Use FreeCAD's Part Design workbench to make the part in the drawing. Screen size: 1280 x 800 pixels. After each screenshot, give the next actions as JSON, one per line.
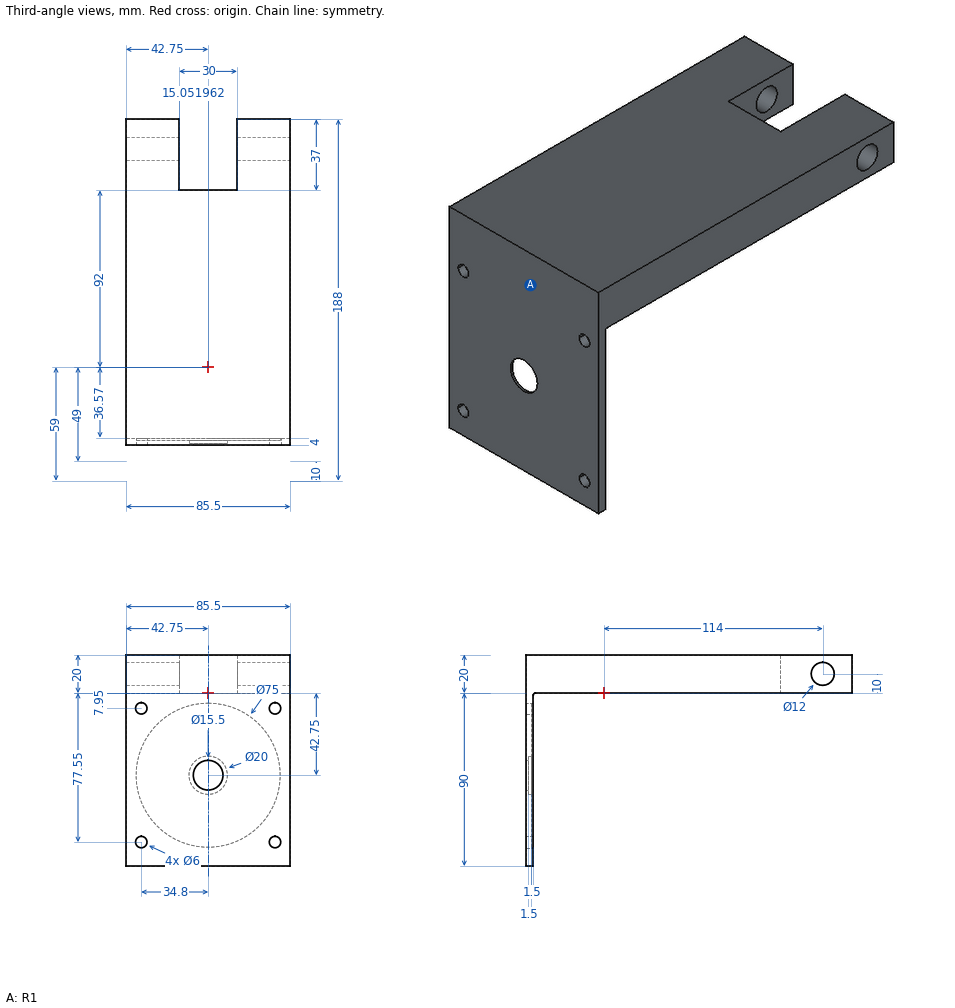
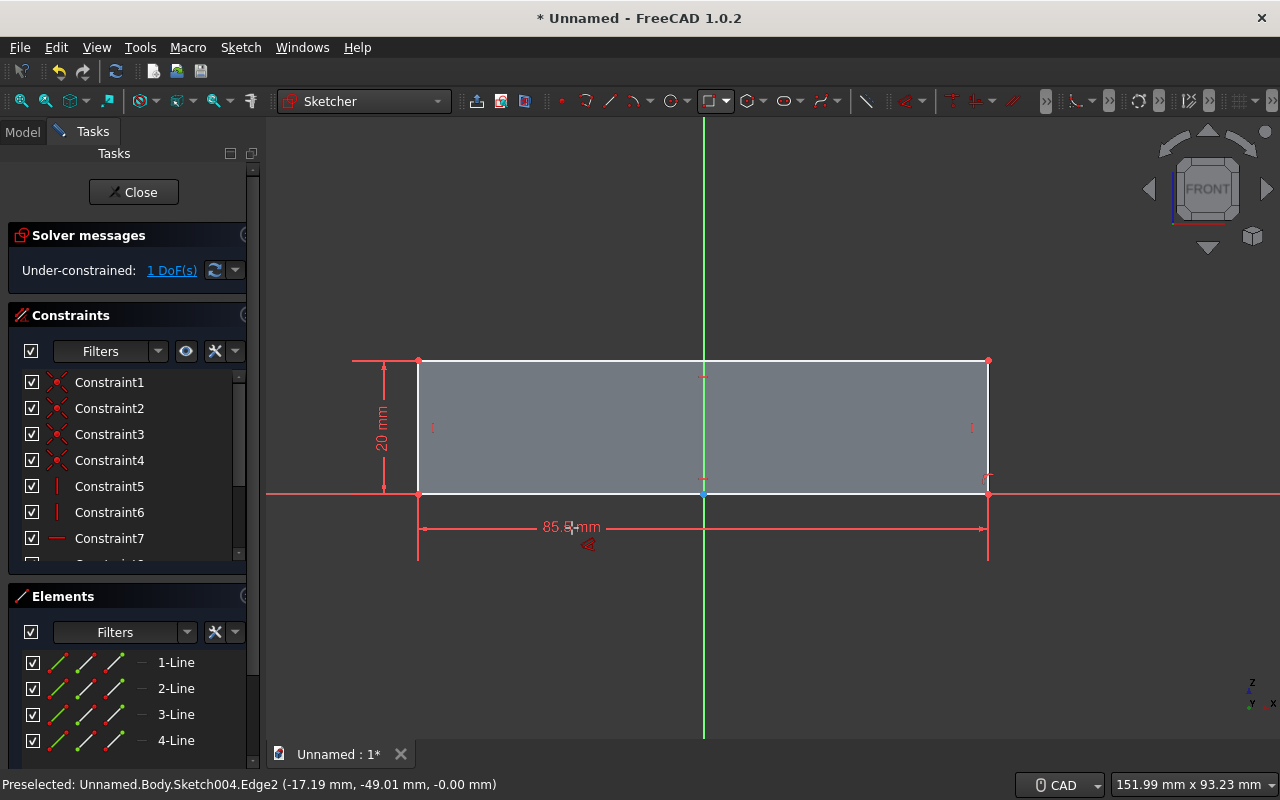
{"action": "left_click", "coordinate": [418, 361]}
{"action": "left_click", "coordinate": [495, 528]}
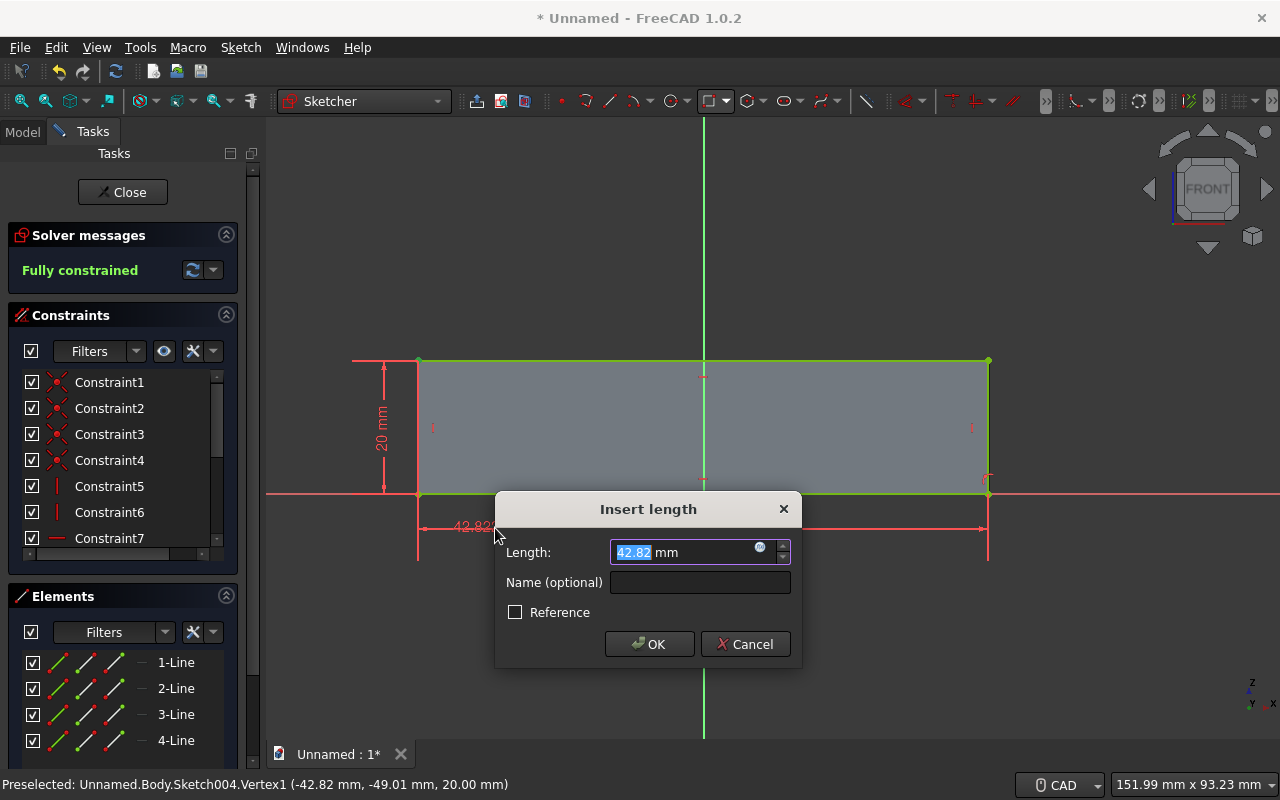
{"action": "type", "text": "42.75"}
{"action": "key", "text": "Return"}
{"action": "key", "text": "Escape"}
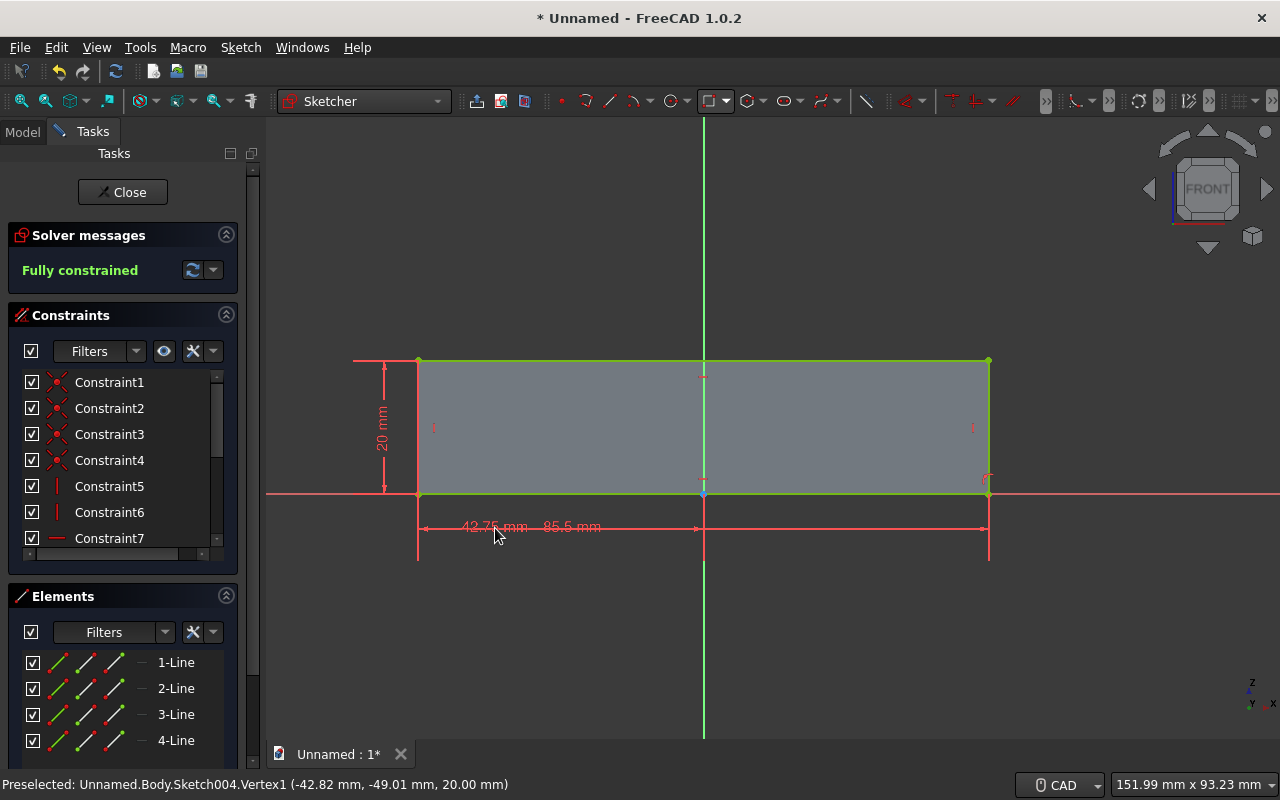
{"action": "left_click", "coordinate": [123, 192]}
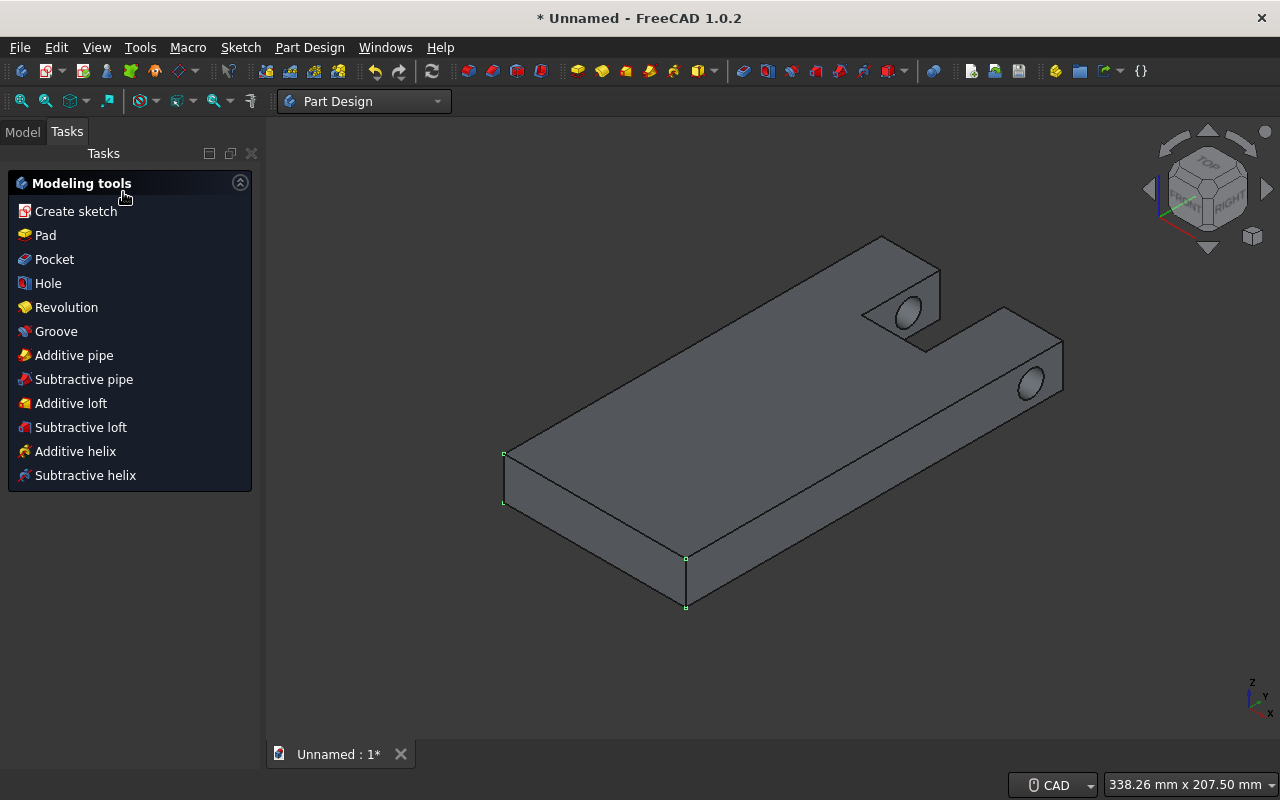
{"action": "left_click", "coordinate": [744, 72]}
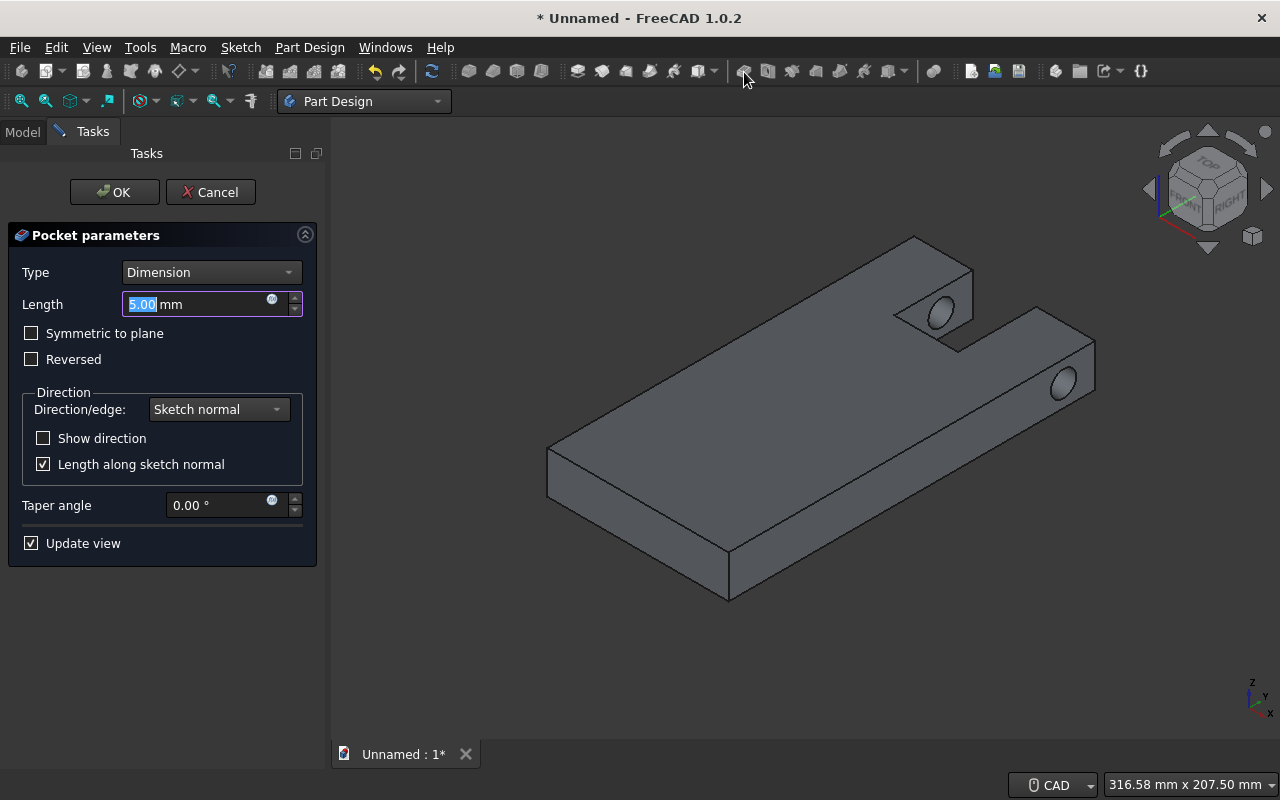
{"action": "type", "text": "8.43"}
{"action": "key", "text": "Tab"}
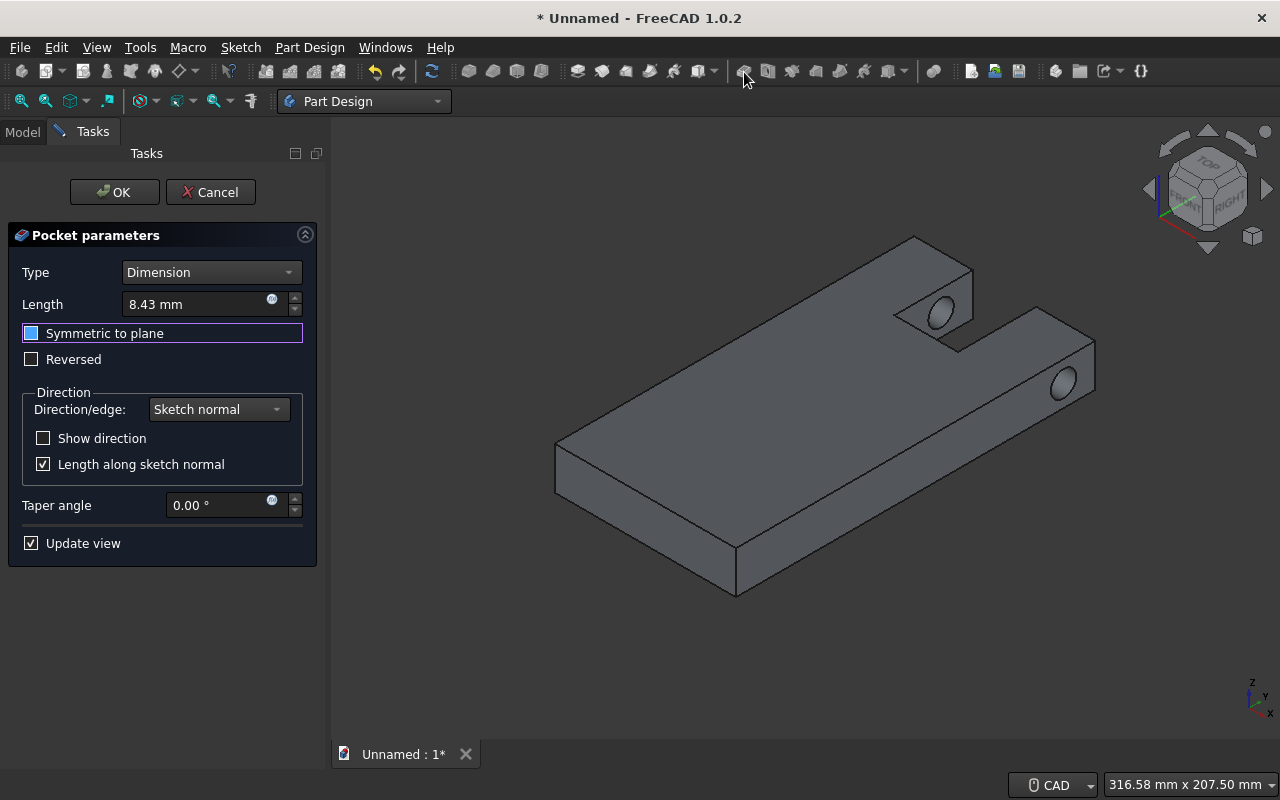
{"action": "left_click", "coordinate": [115, 192]}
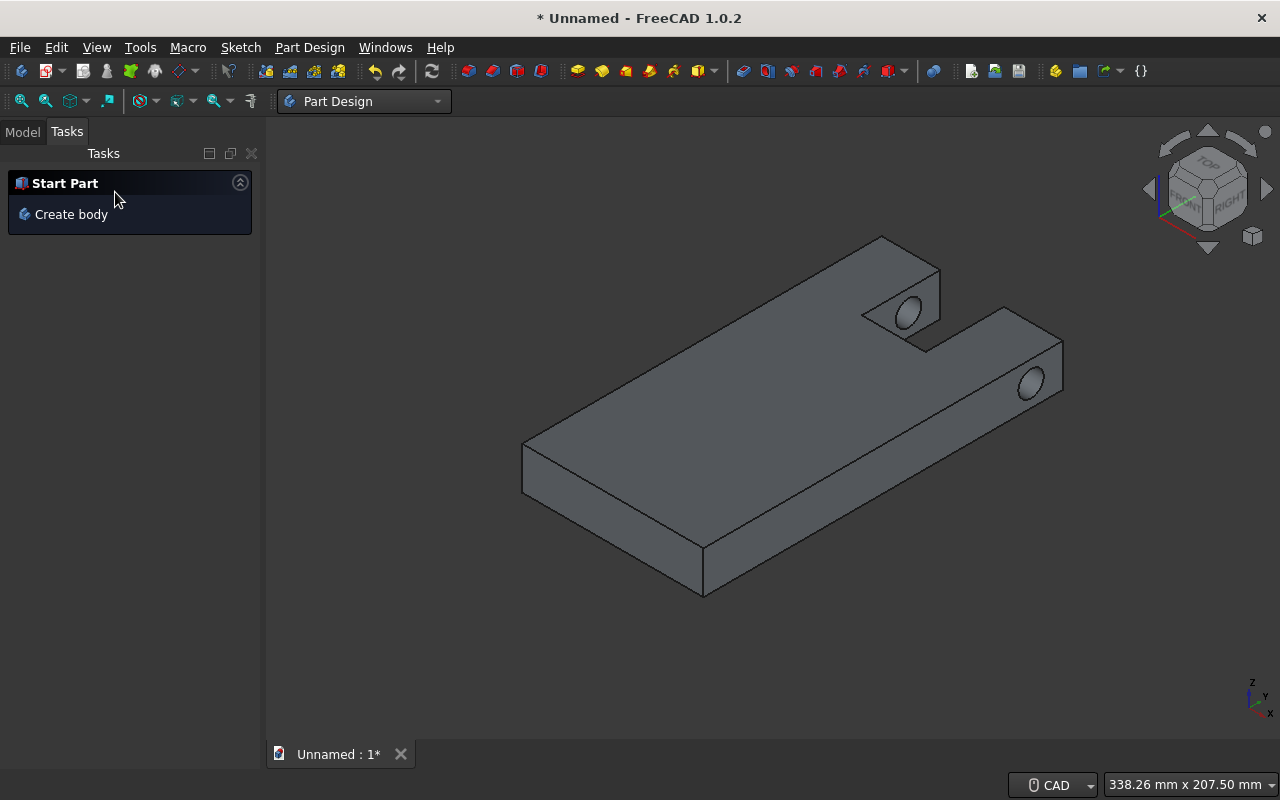
{"action": "left_click", "coordinate": [46, 72]}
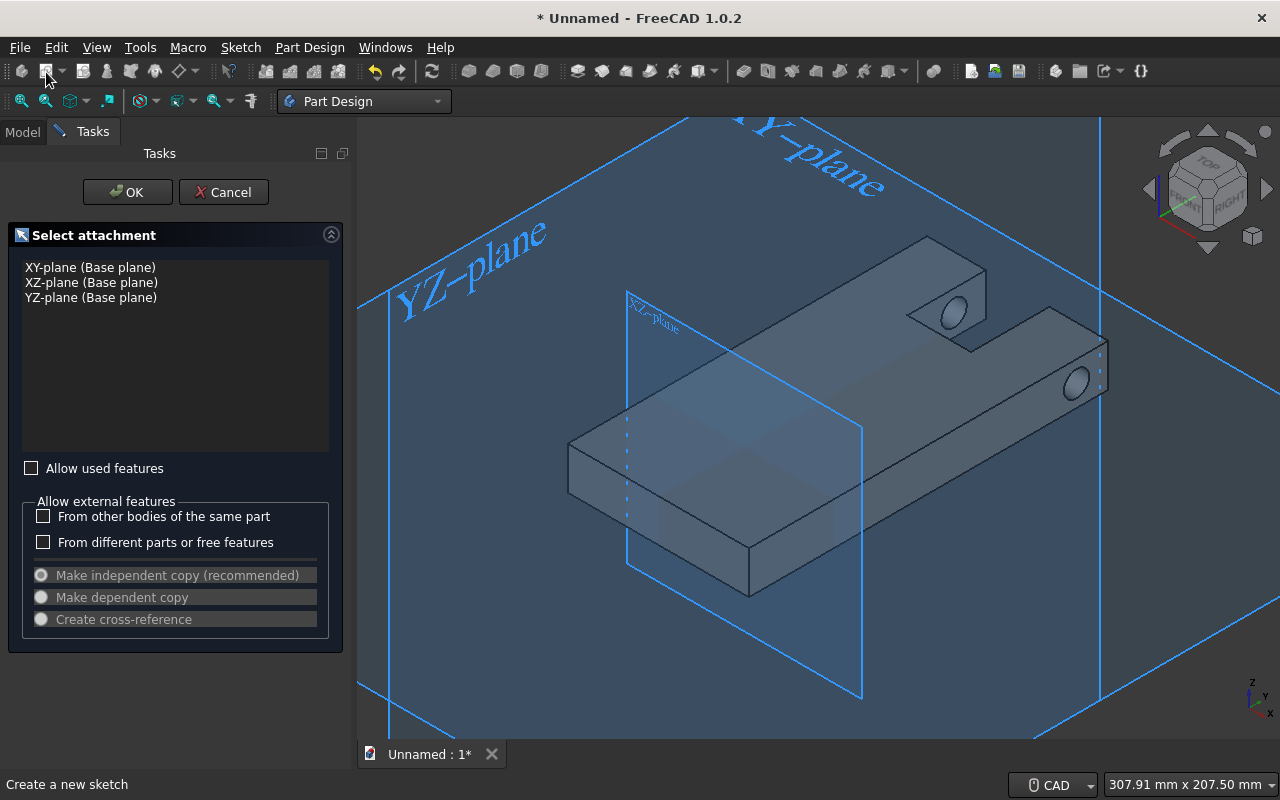
{"action": "left_click", "coordinate": [82, 268]}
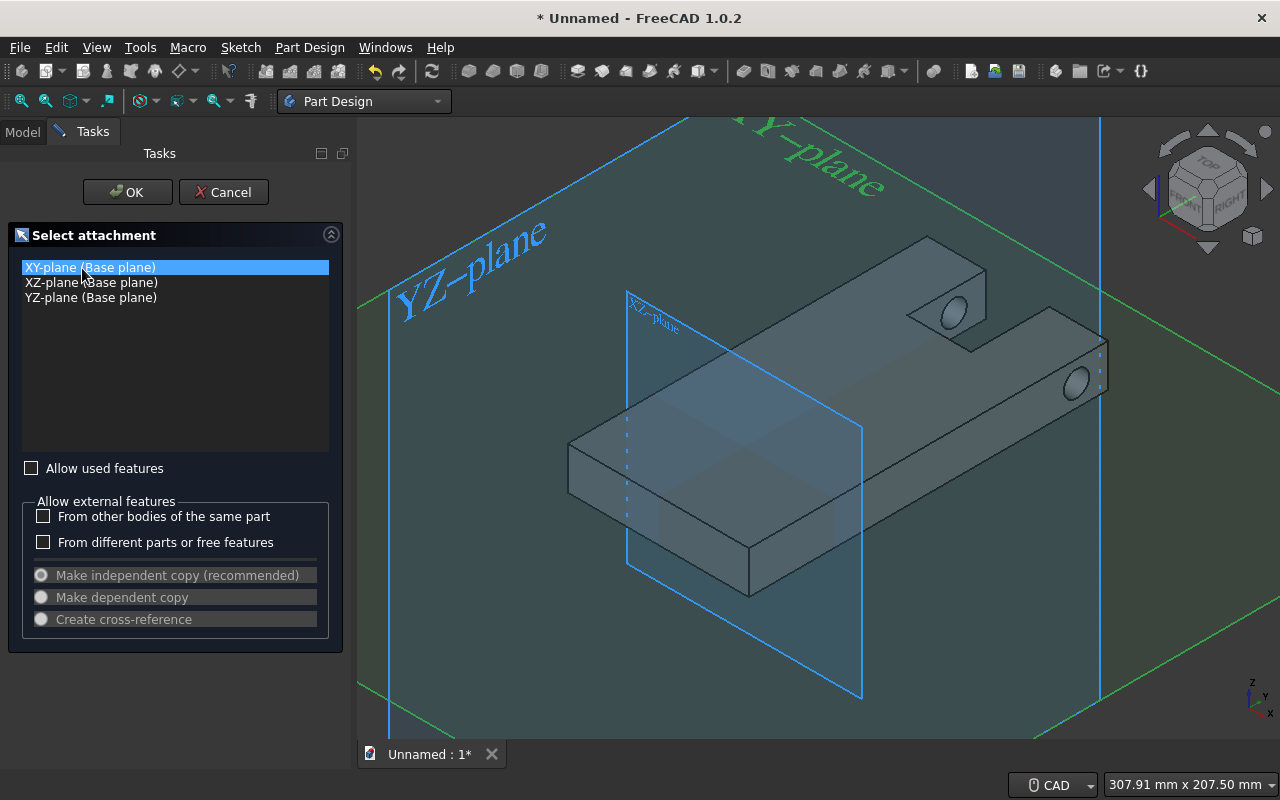
{"action": "left_click", "coordinate": [128, 192]}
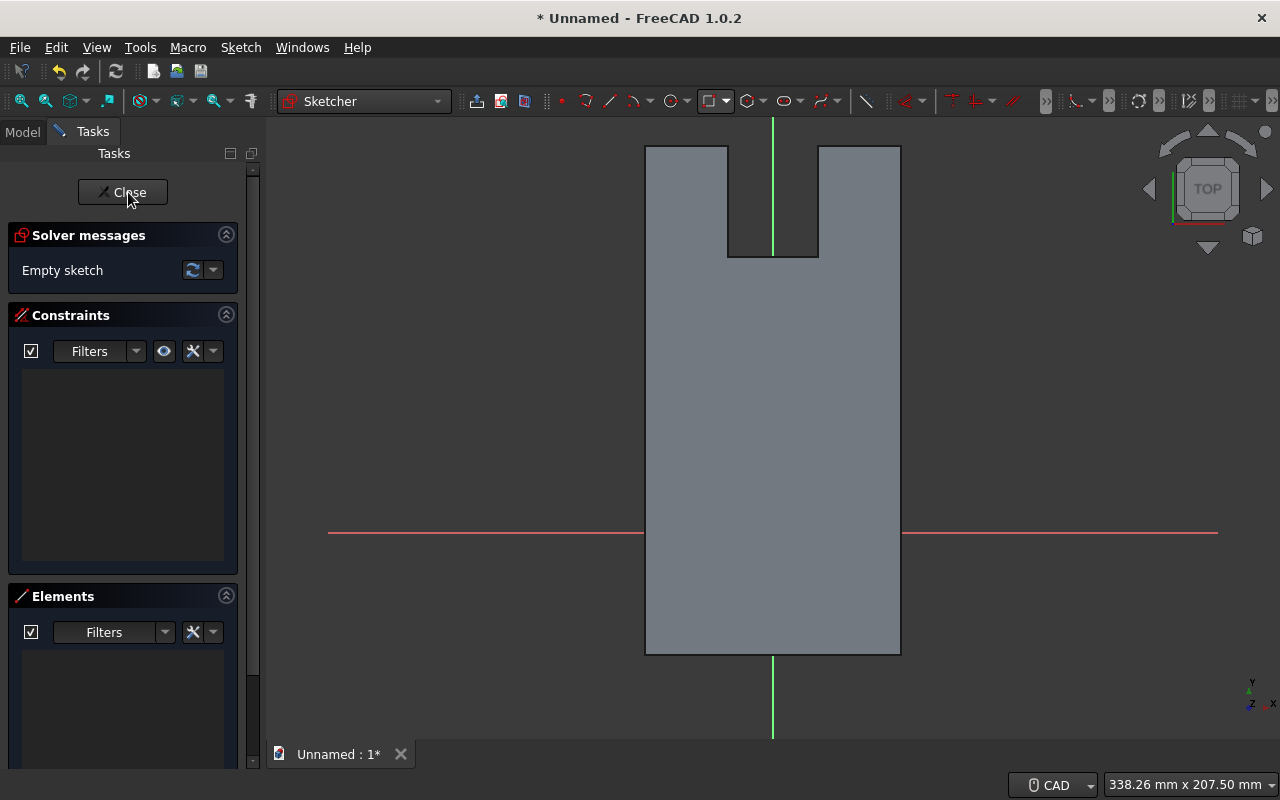
{"action": "key", "text": "q s"}